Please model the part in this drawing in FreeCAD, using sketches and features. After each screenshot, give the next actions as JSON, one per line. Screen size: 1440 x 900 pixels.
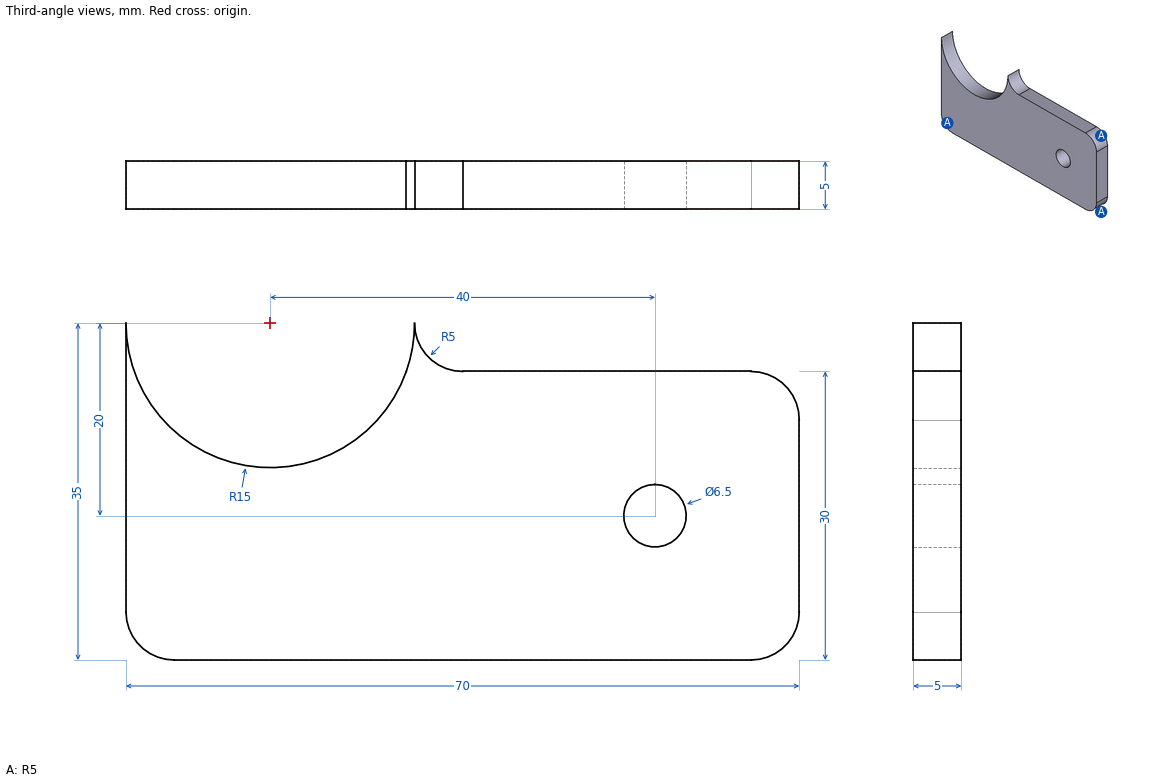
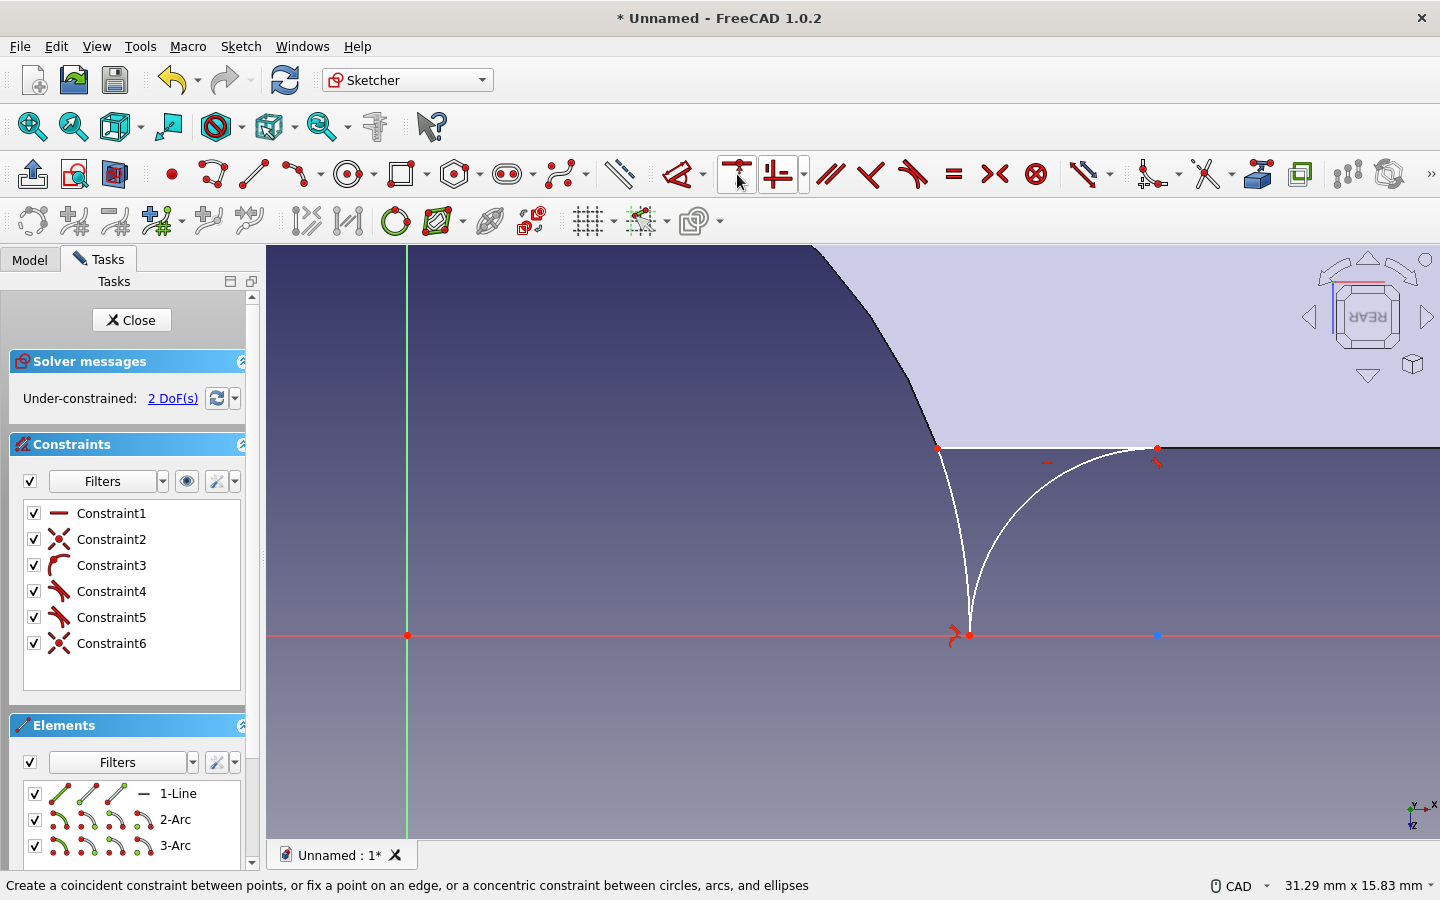
{"action": "left_click", "coordinate": [676, 174]}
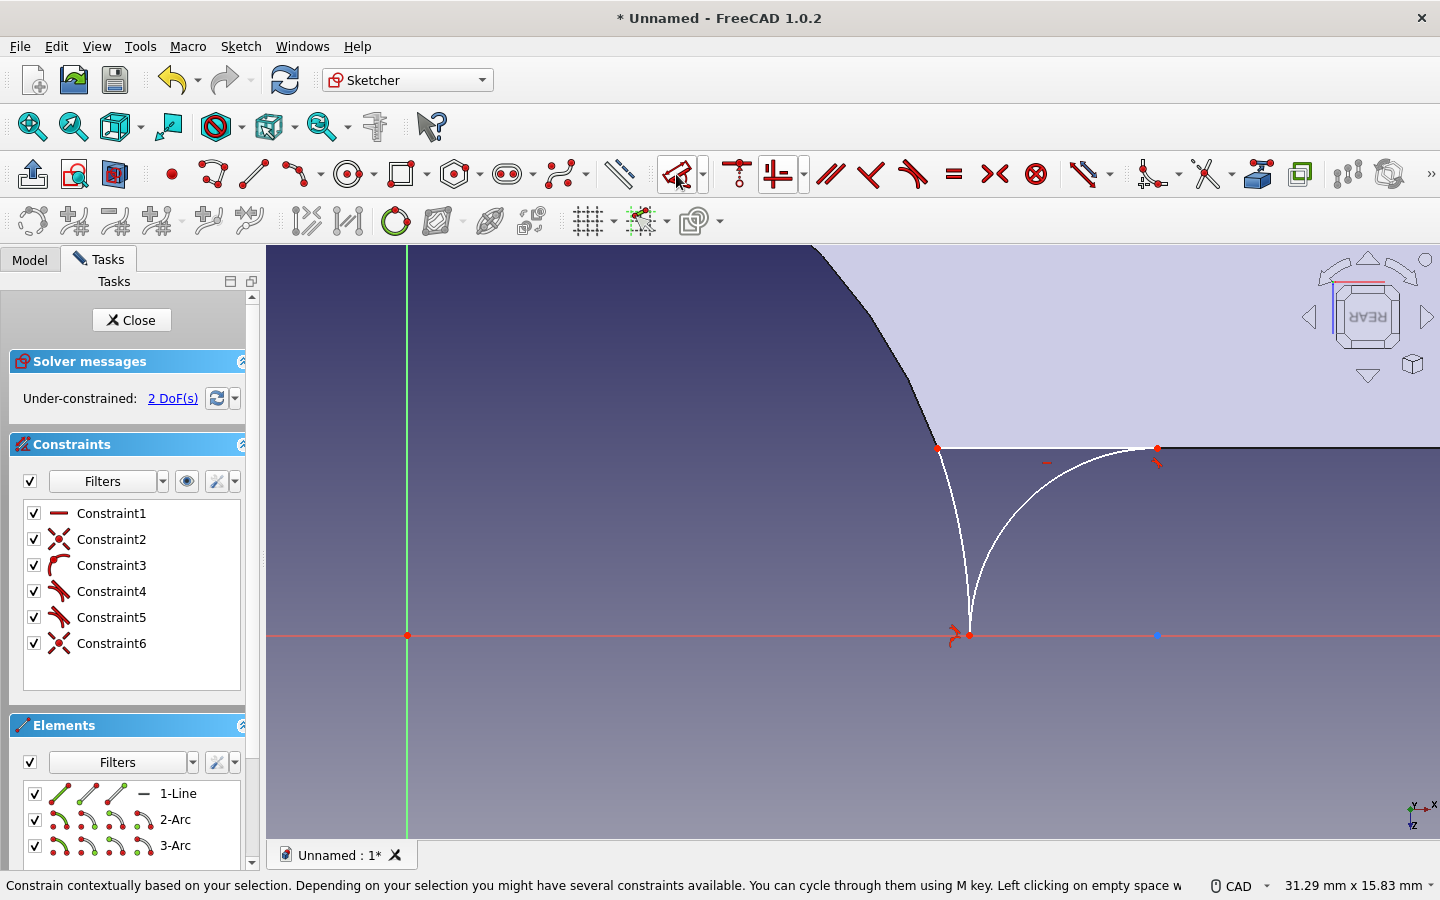
{"action": "left_click", "coordinate": [967, 579]}
{"action": "left_click", "coordinate": [999, 576]}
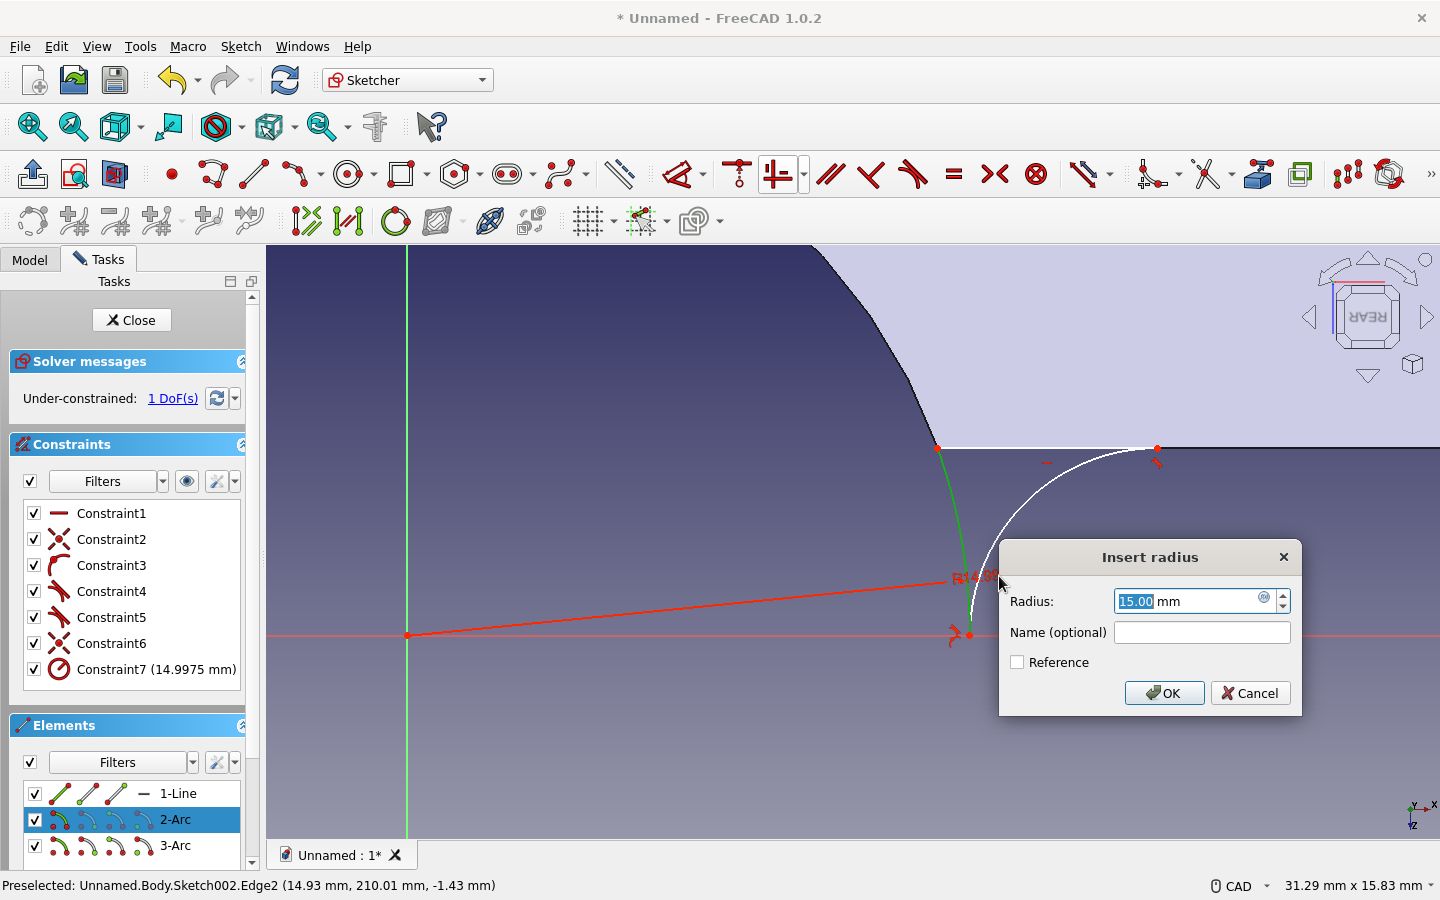
{"action": "type", "text": "15"}
{"action": "key", "text": "Return"}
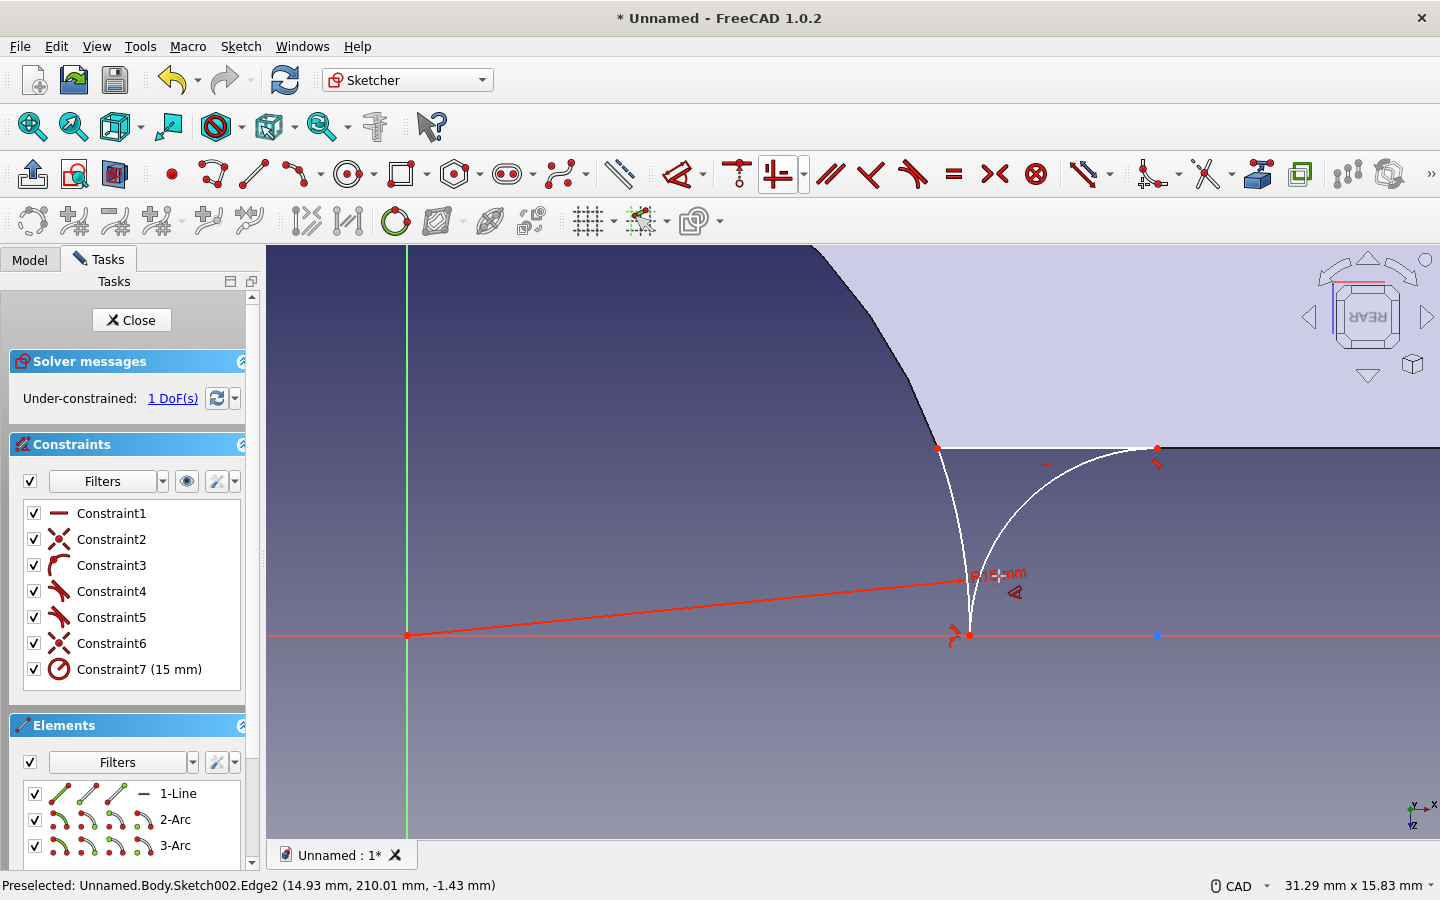
{"action": "left_click", "coordinate": [1073, 469]}
{"action": "left_click", "coordinate": [1164, 417]}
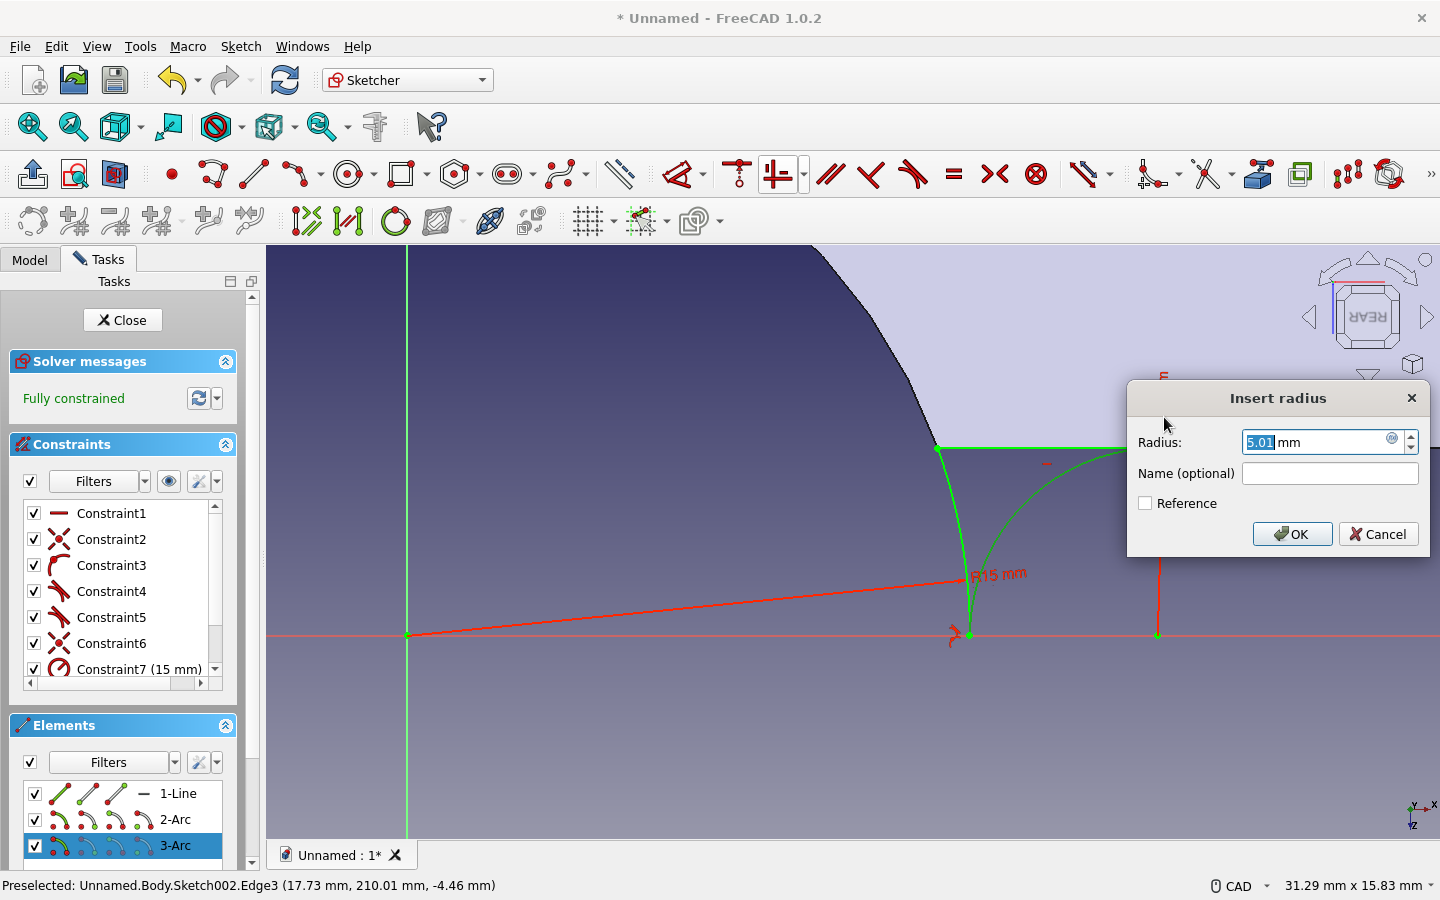
{"action": "type", "text": "5"}
{"action": "key", "text": "Return"}
{"action": "key", "text": "Escape"}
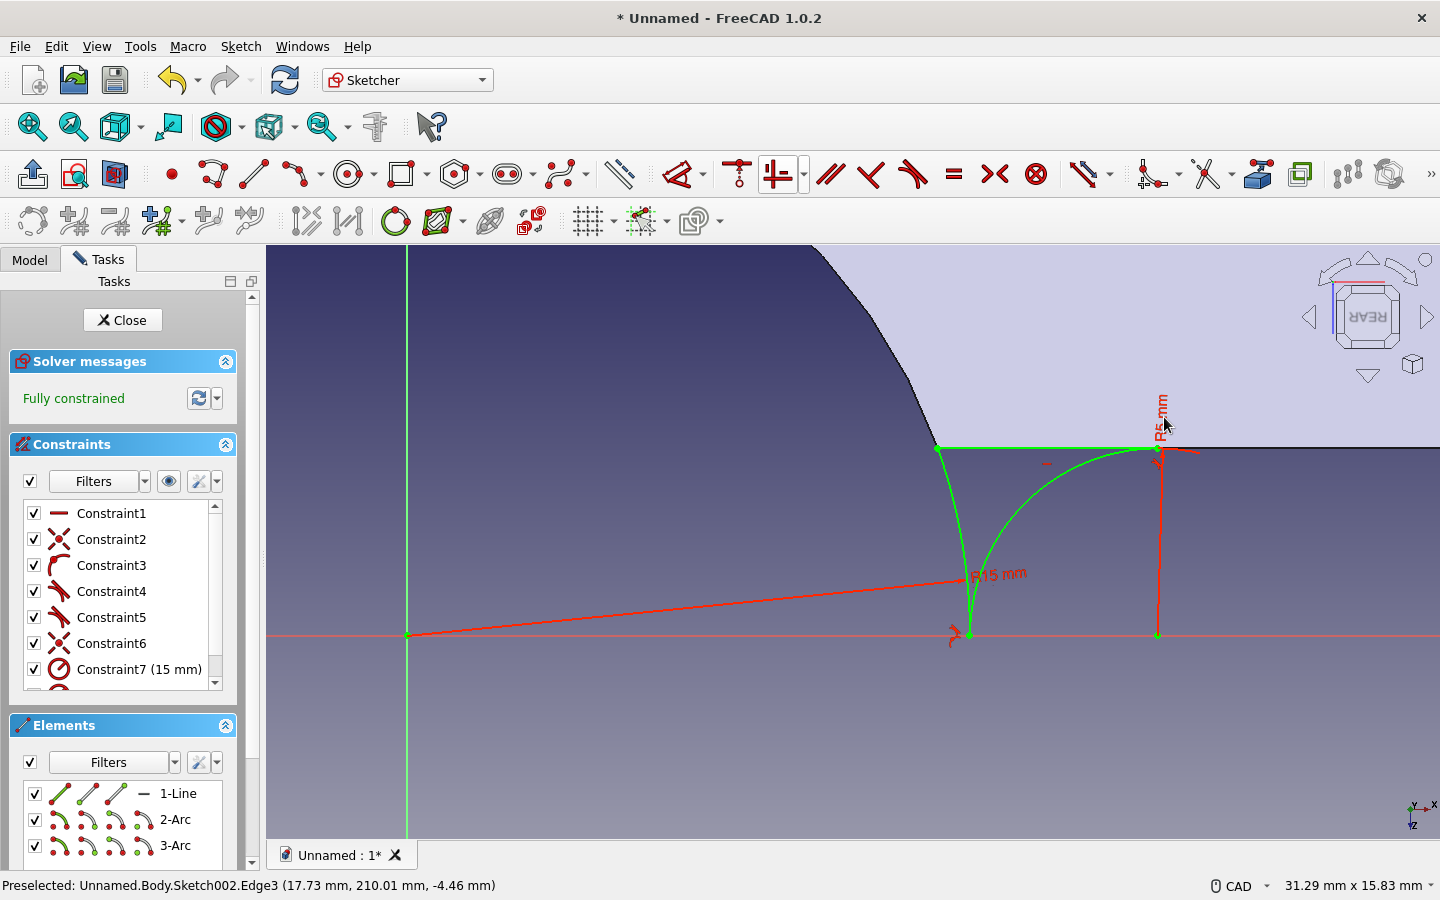
{"action": "left_click", "coordinate": [123, 320]}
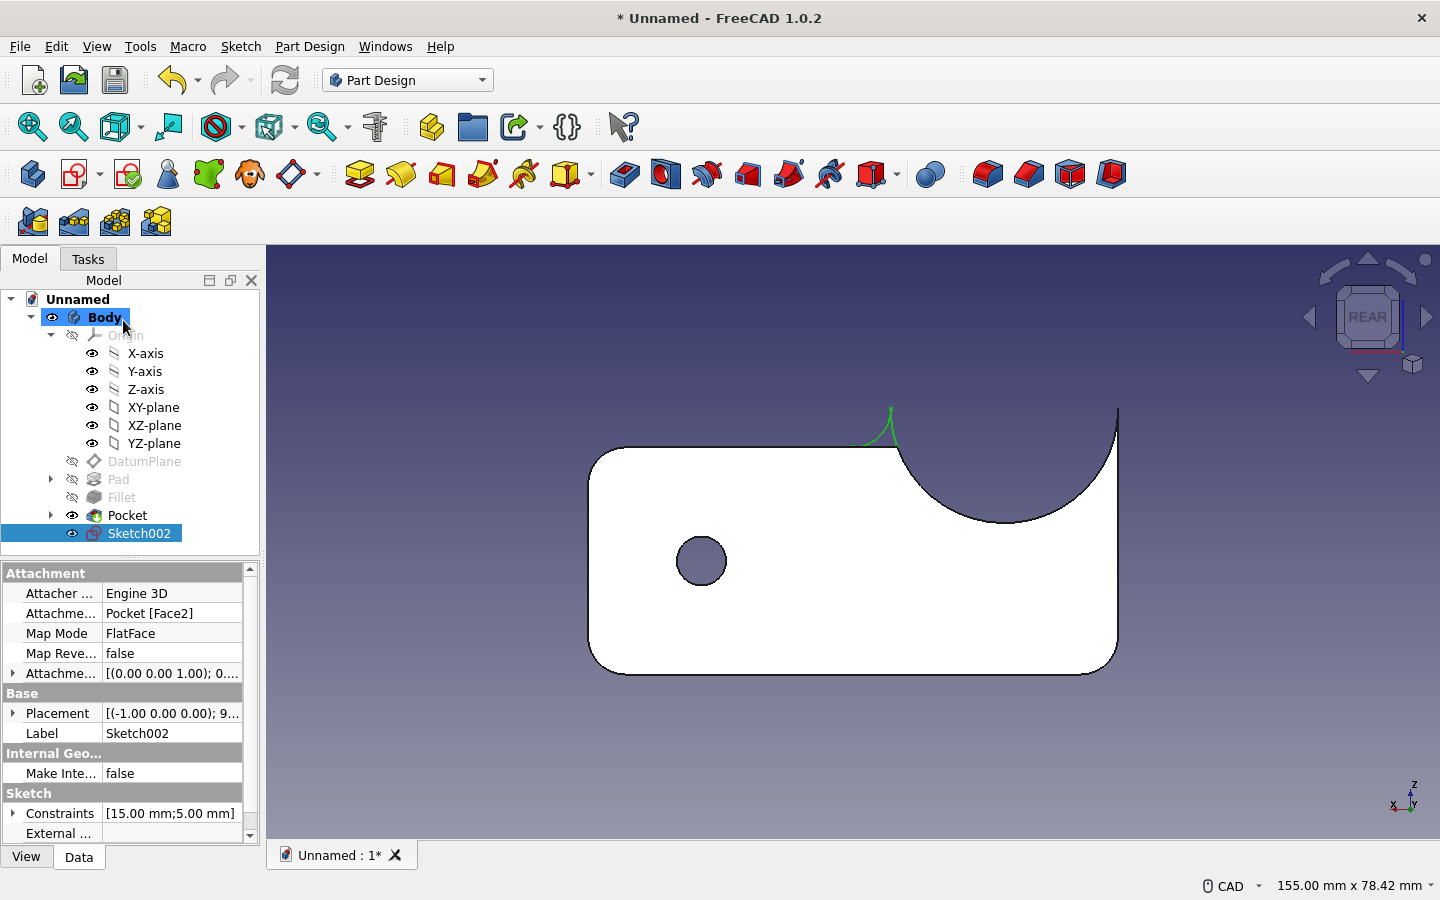
{"action": "left_click", "coordinate": [360, 174]}